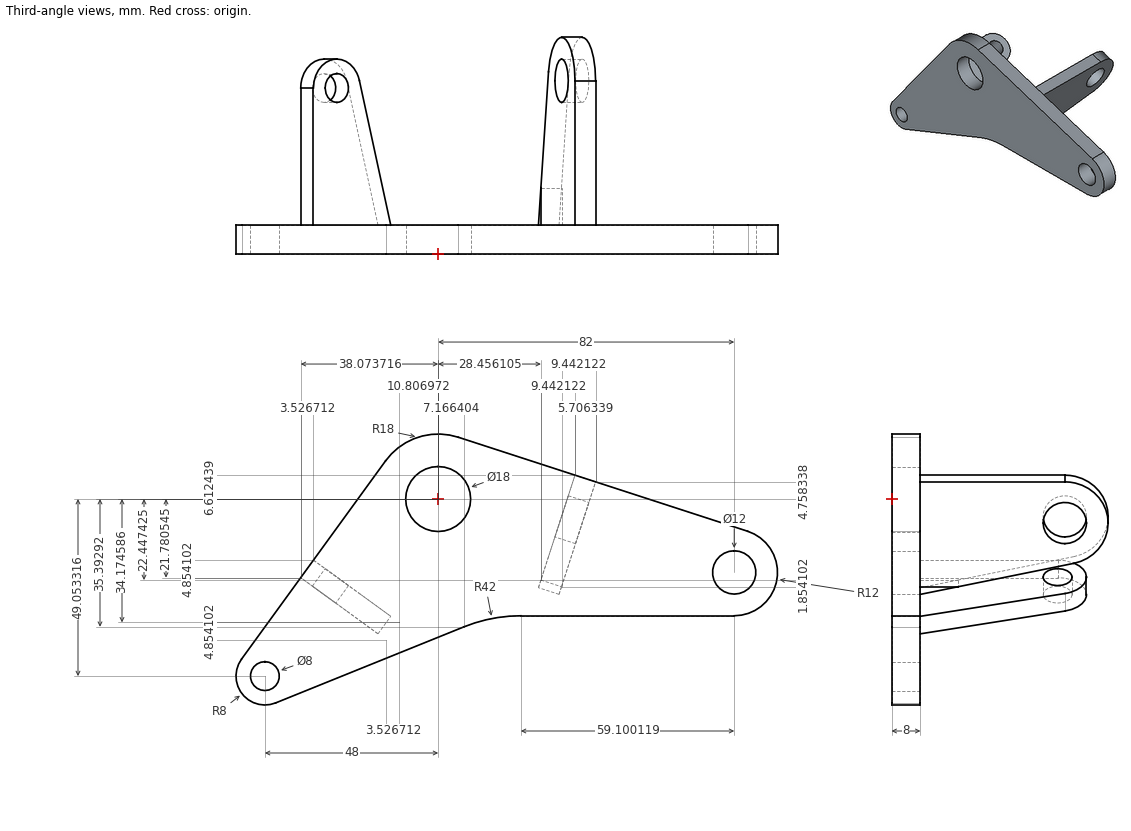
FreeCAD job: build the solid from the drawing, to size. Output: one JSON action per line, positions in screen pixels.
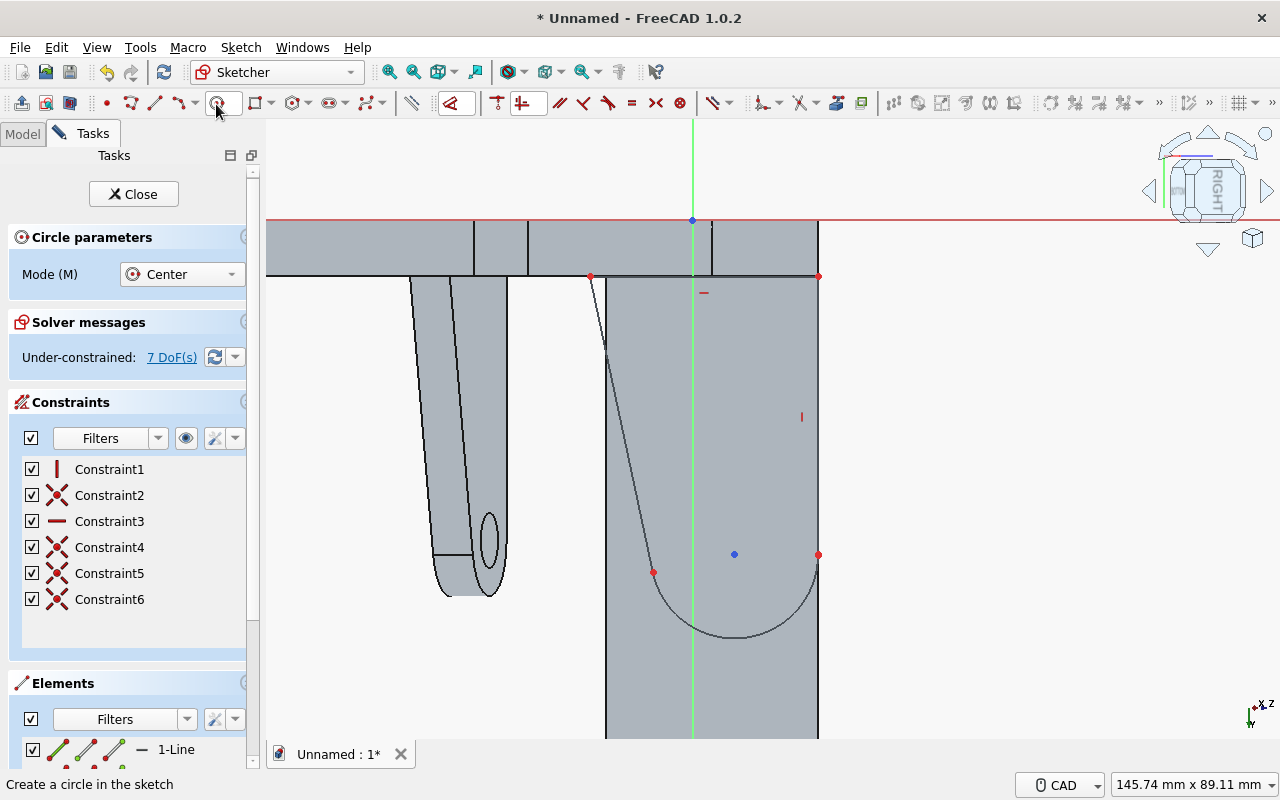
{"action": "left_click", "coordinate": [735, 554]}
{"action": "mouse_move", "coordinate": [764, 525]}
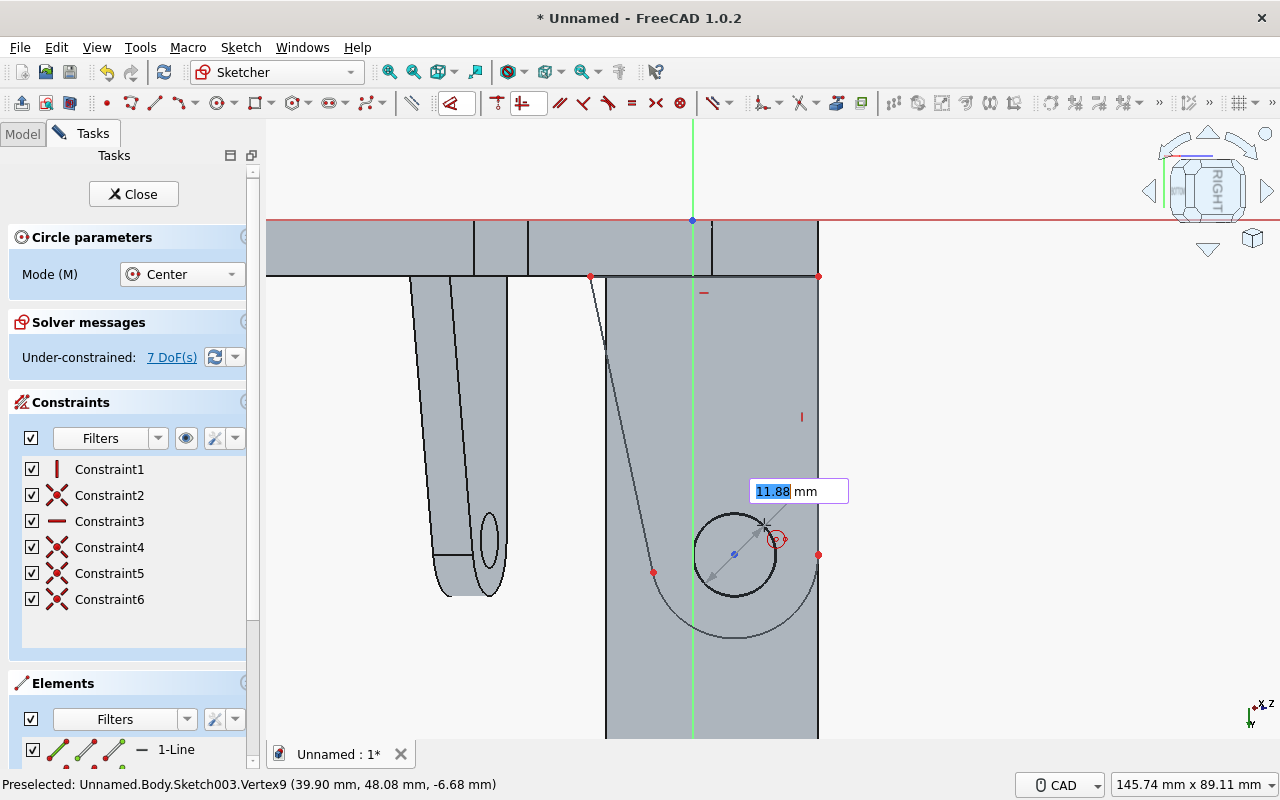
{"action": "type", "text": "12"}
{"action": "key", "text": "Return"}
{"action": "key", "text": "Escape"}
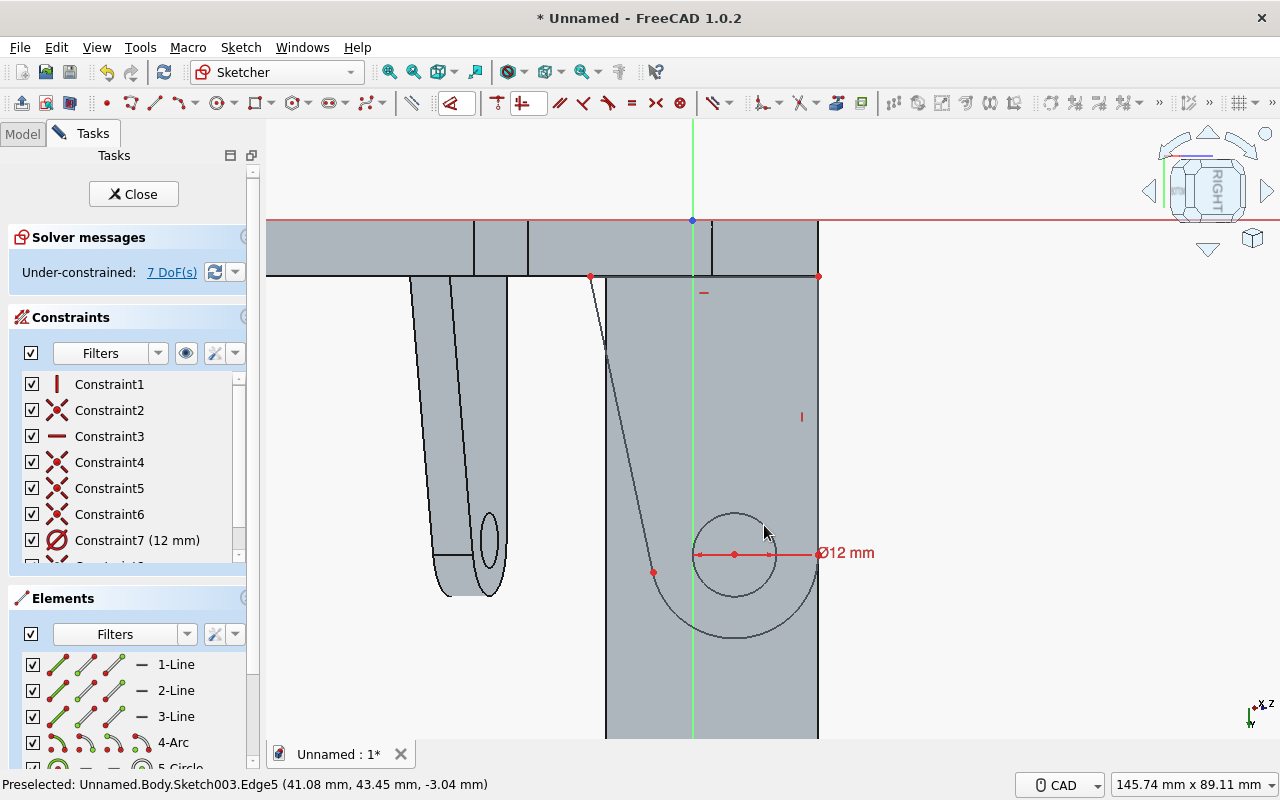
{"action": "left_click", "coordinate": [818, 472]}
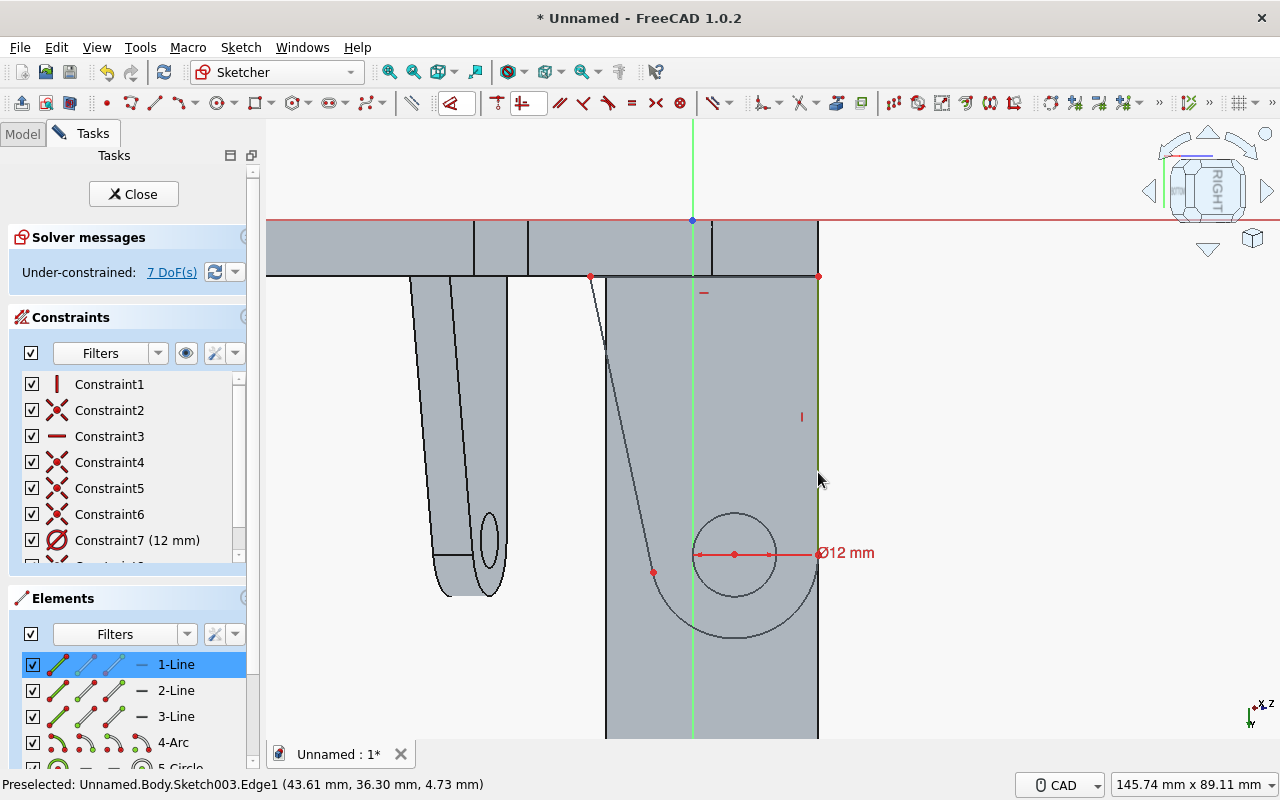
{"action": "left_click", "coordinate": [696, 629]}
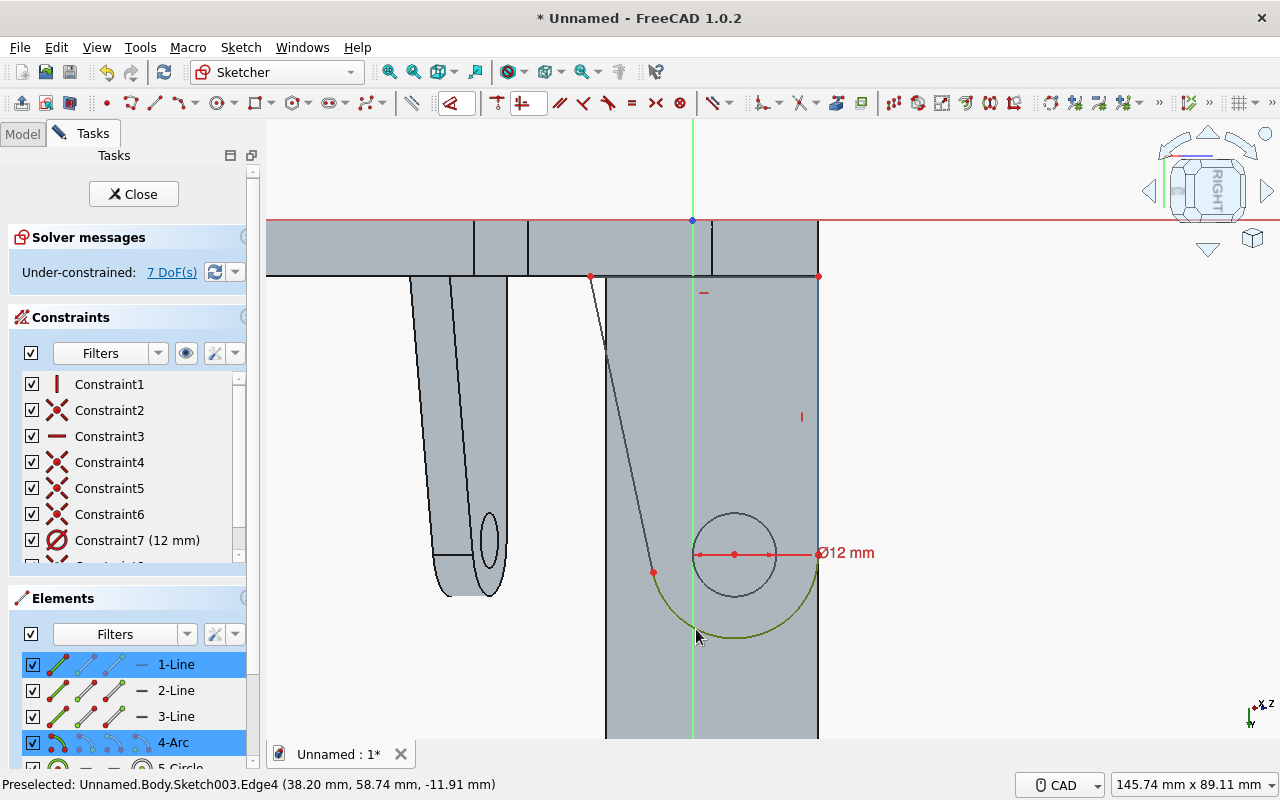
{"action": "key", "text": "t"}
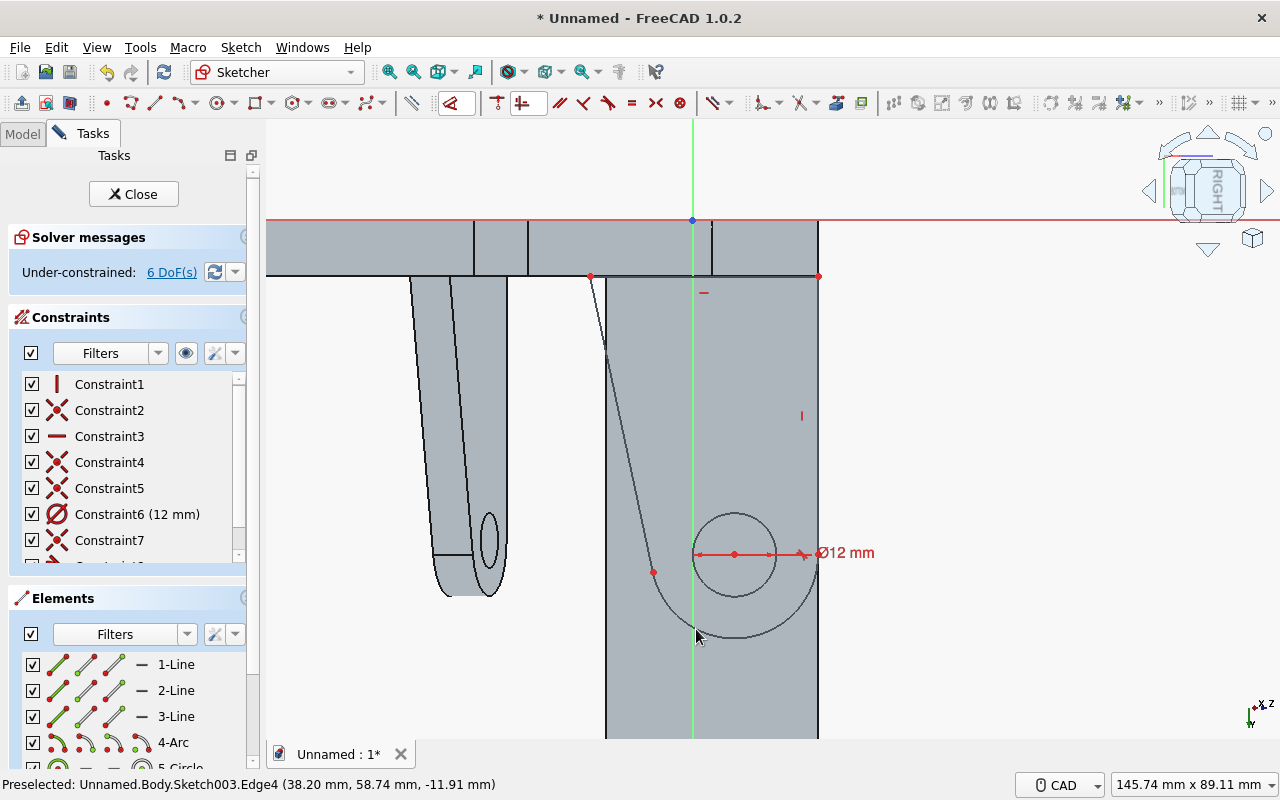
{"action": "left_click", "coordinate": [609, 366]}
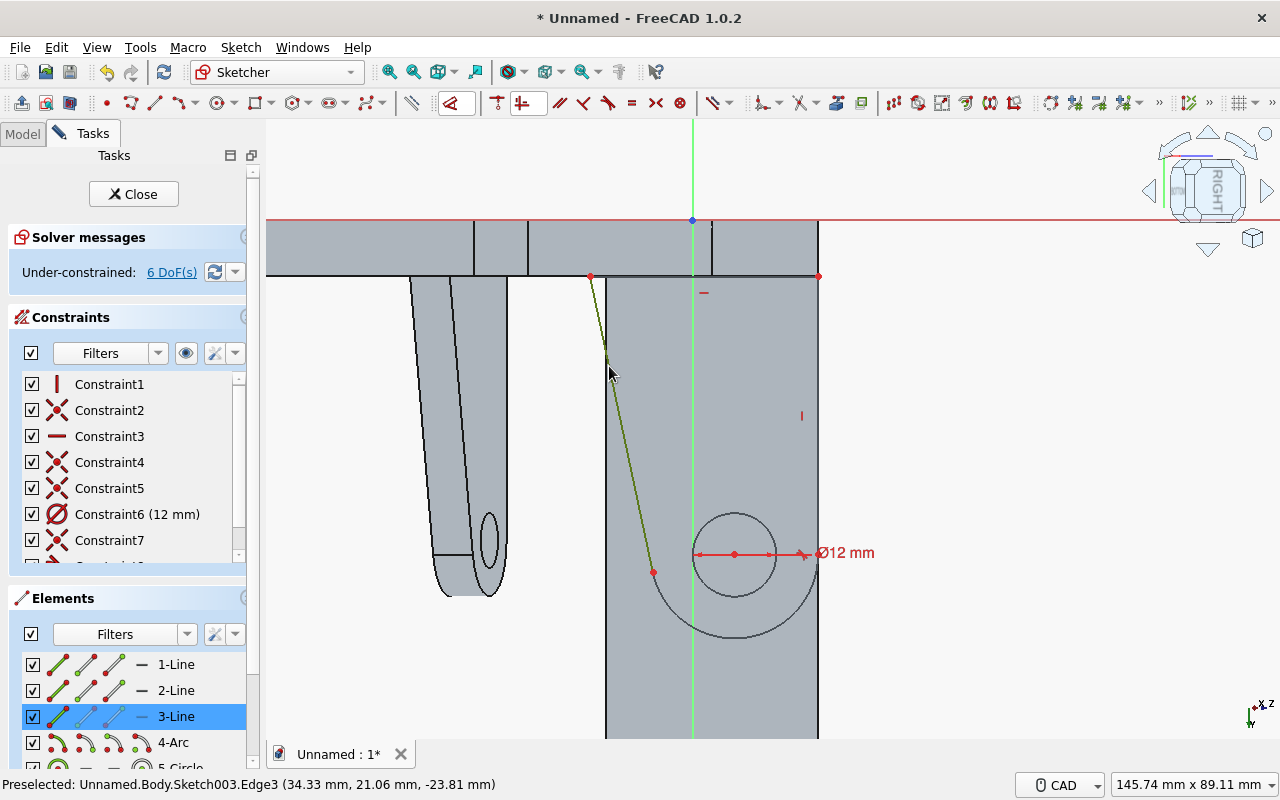
{"action": "left_click", "coordinate": [696, 629]}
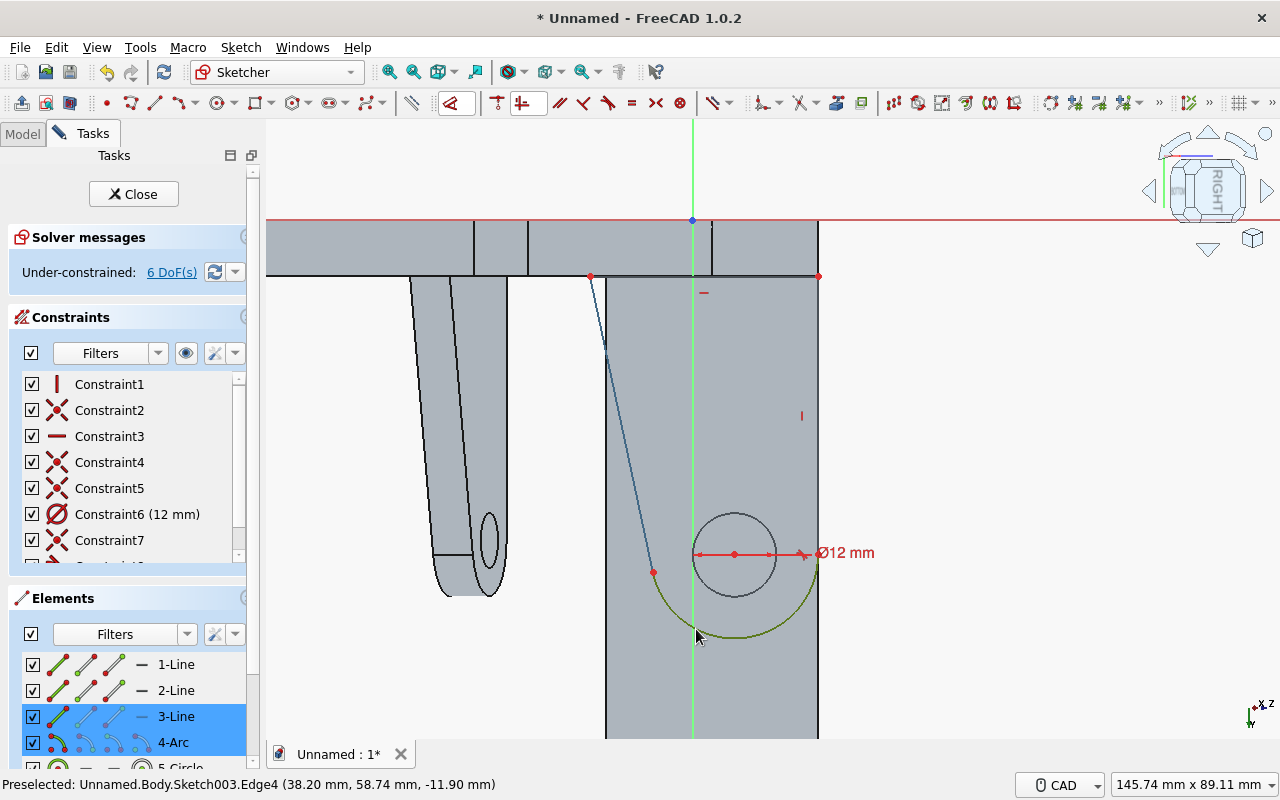
{"action": "left_click", "coordinate": [608, 104]}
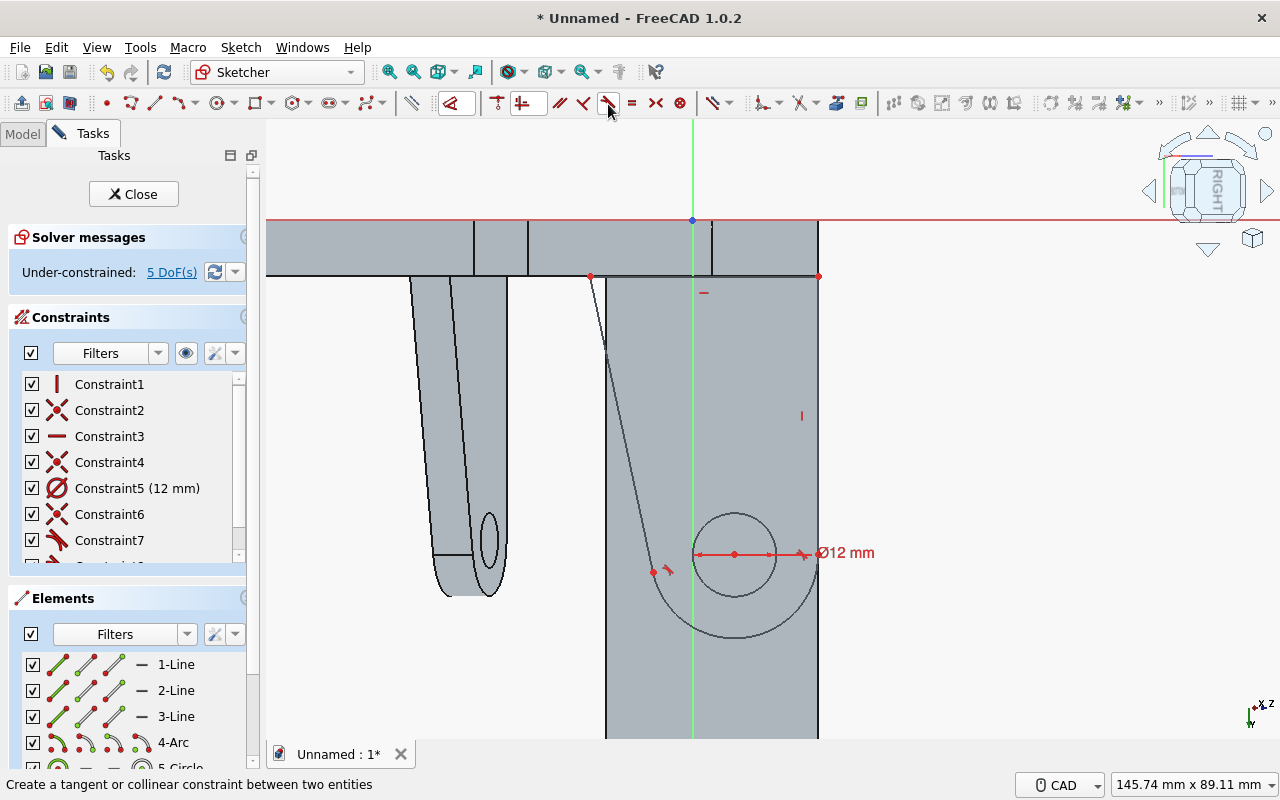
{"action": "left_click", "coordinate": [696, 629]}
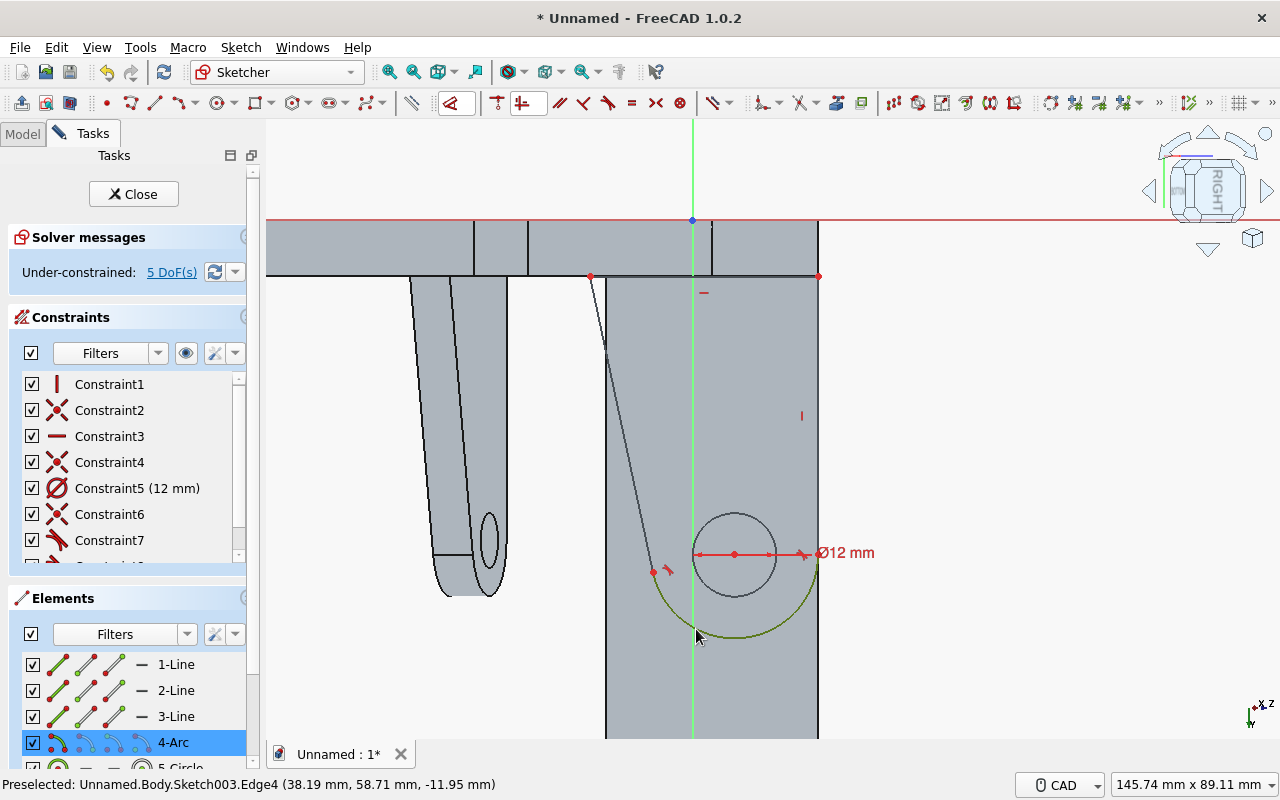
{"action": "left_click", "coordinate": [470, 104]}